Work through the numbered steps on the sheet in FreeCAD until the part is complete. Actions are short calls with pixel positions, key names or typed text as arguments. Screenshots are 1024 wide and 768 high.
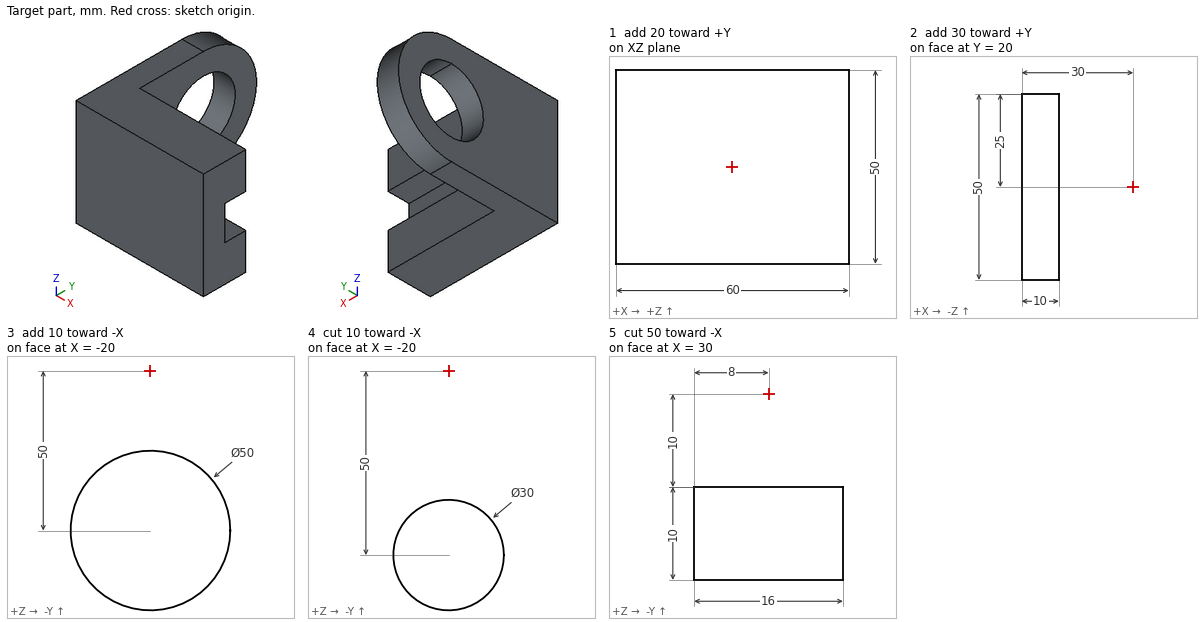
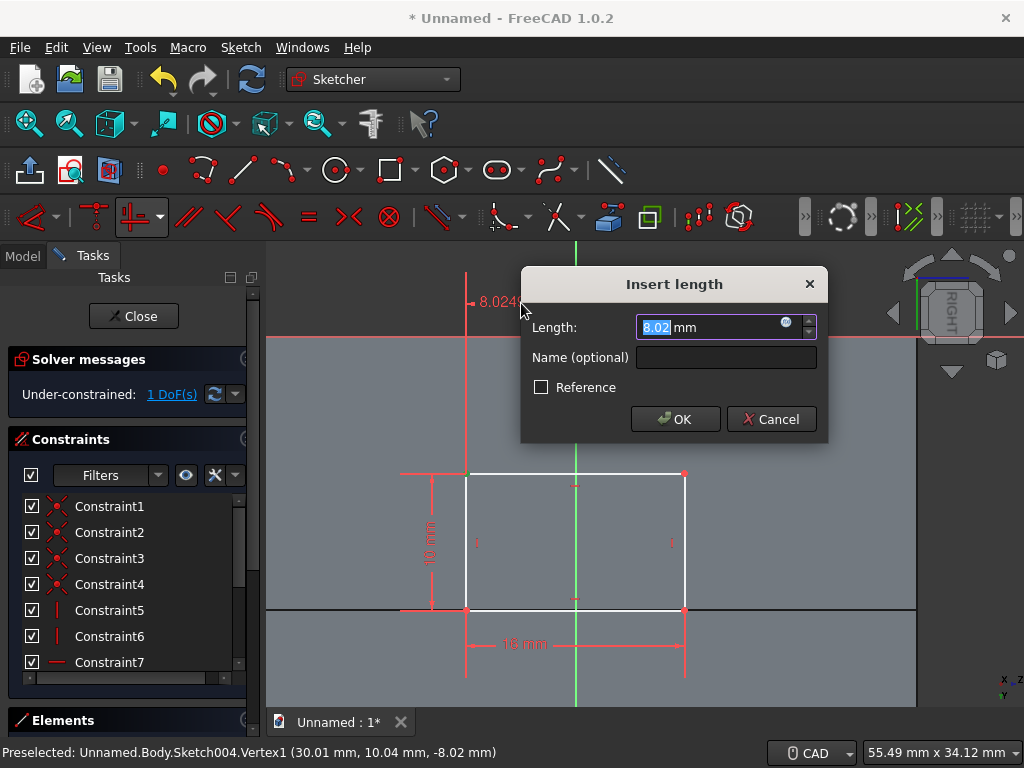
text(8)
key(Return)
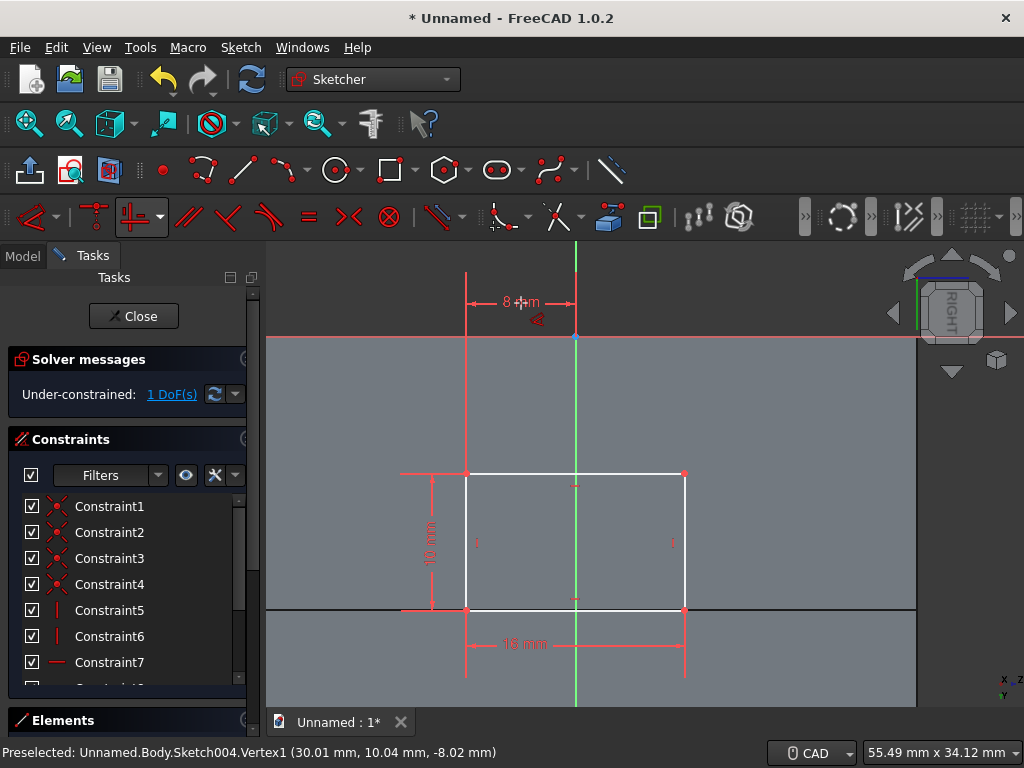
click(466, 474)
click(432, 405)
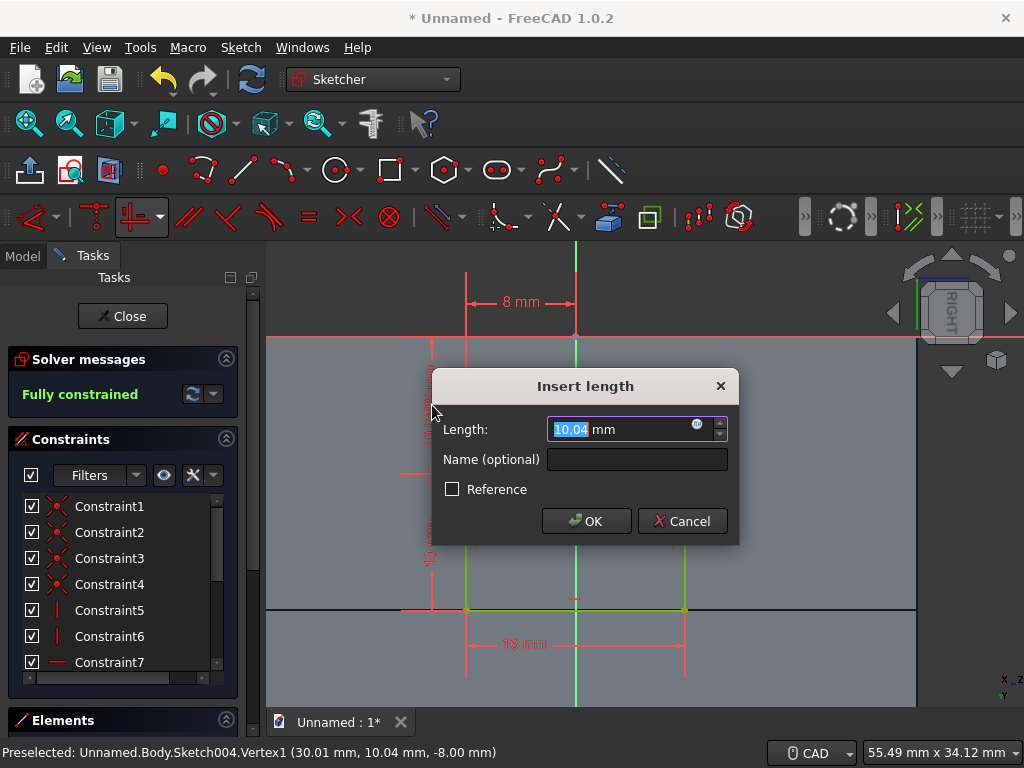
text(10)
key(Return)
key(Escape)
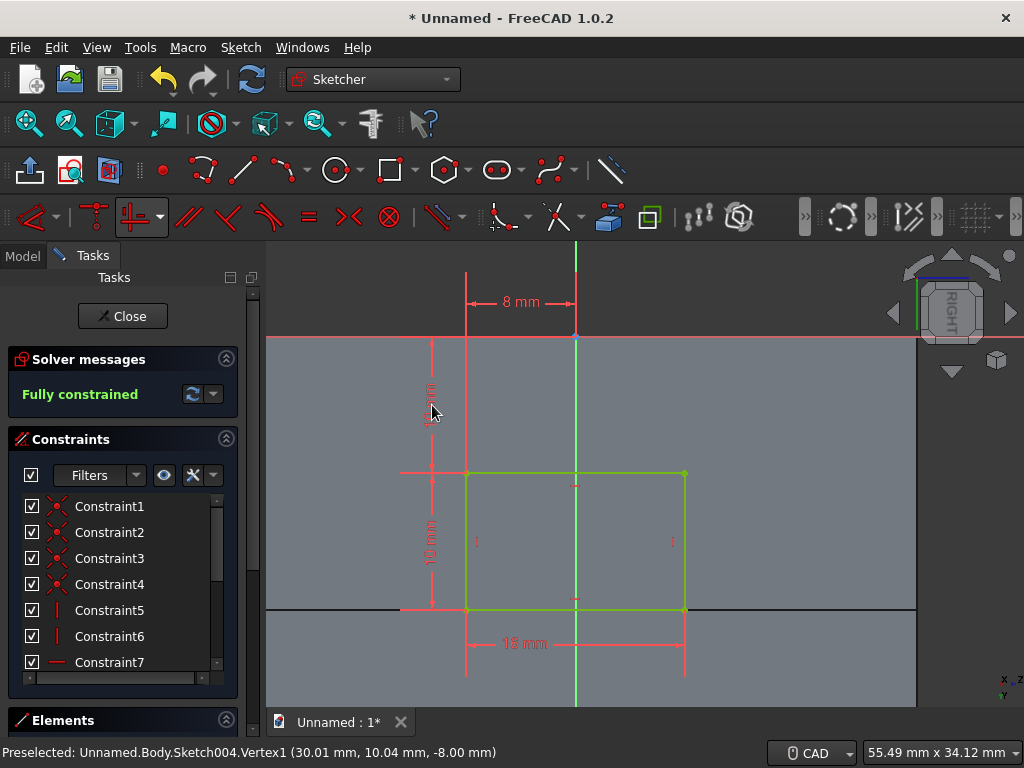
click(123, 316)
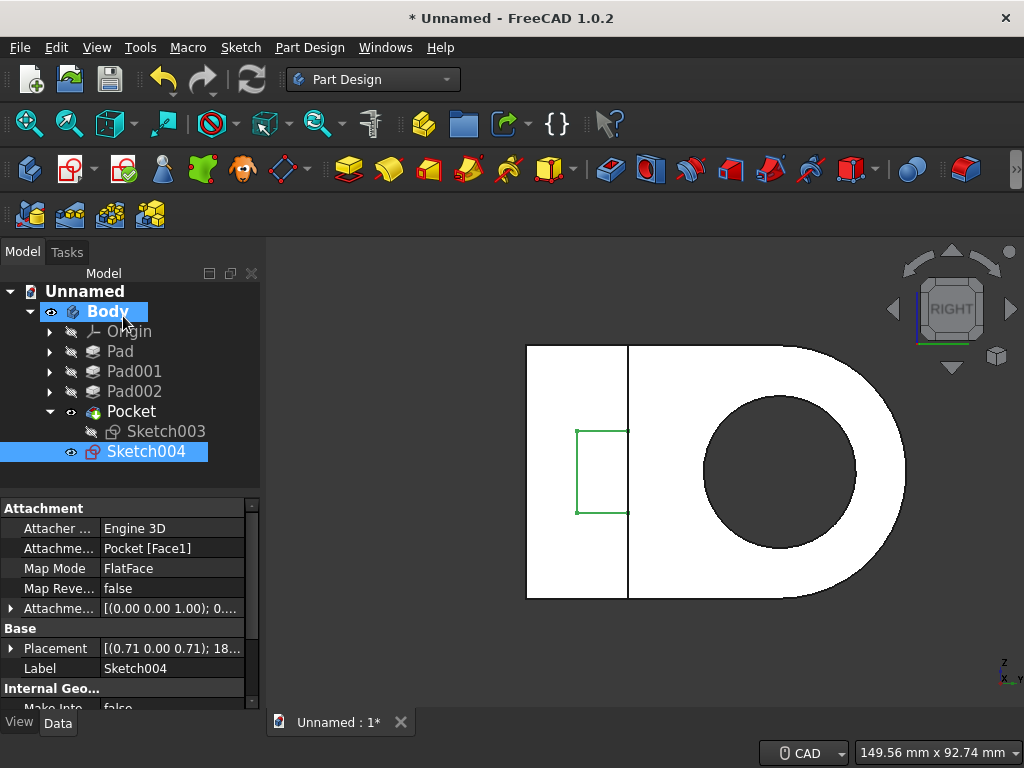
click(612, 170)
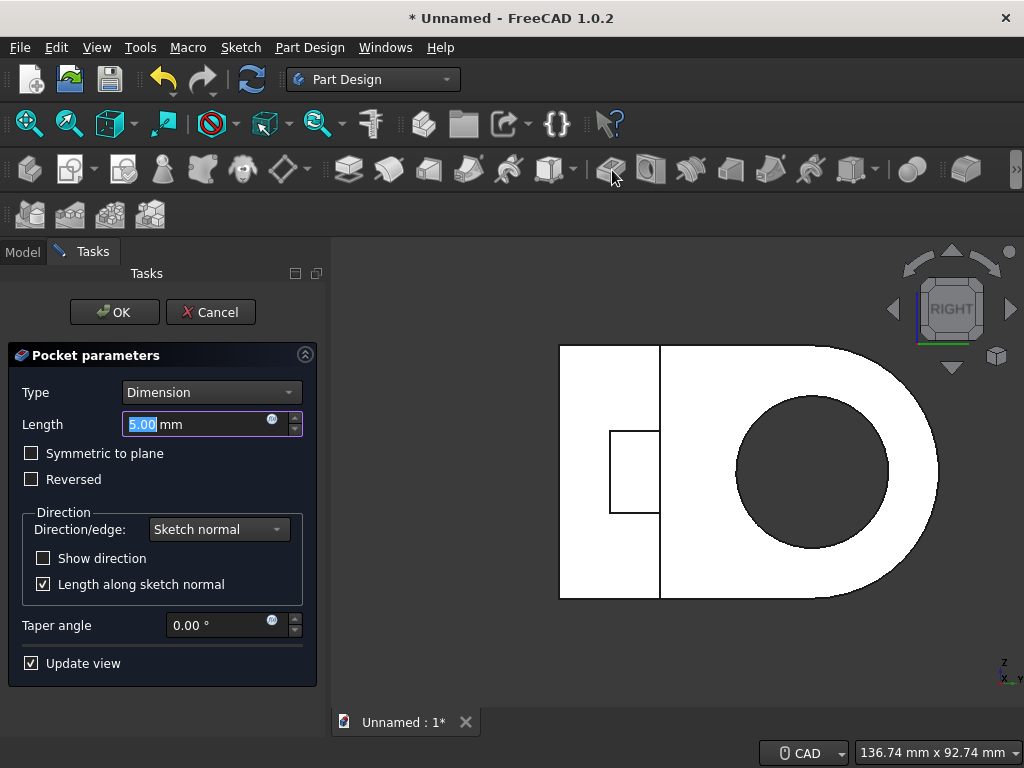
text(50)
key(Tab)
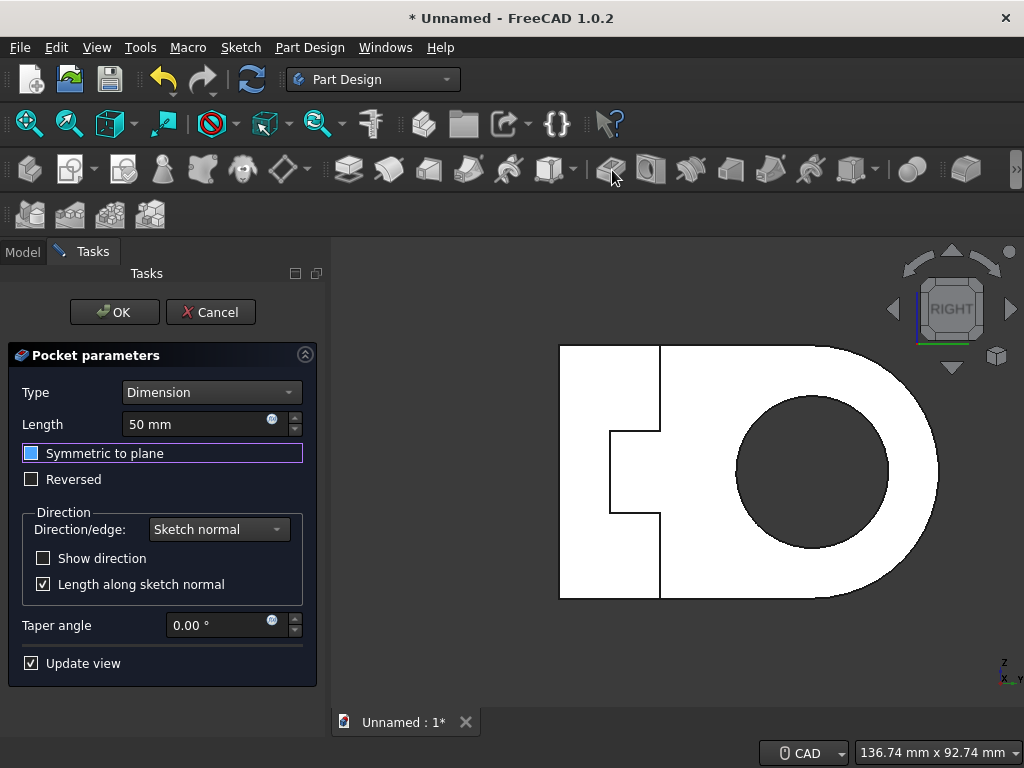
click(115, 312)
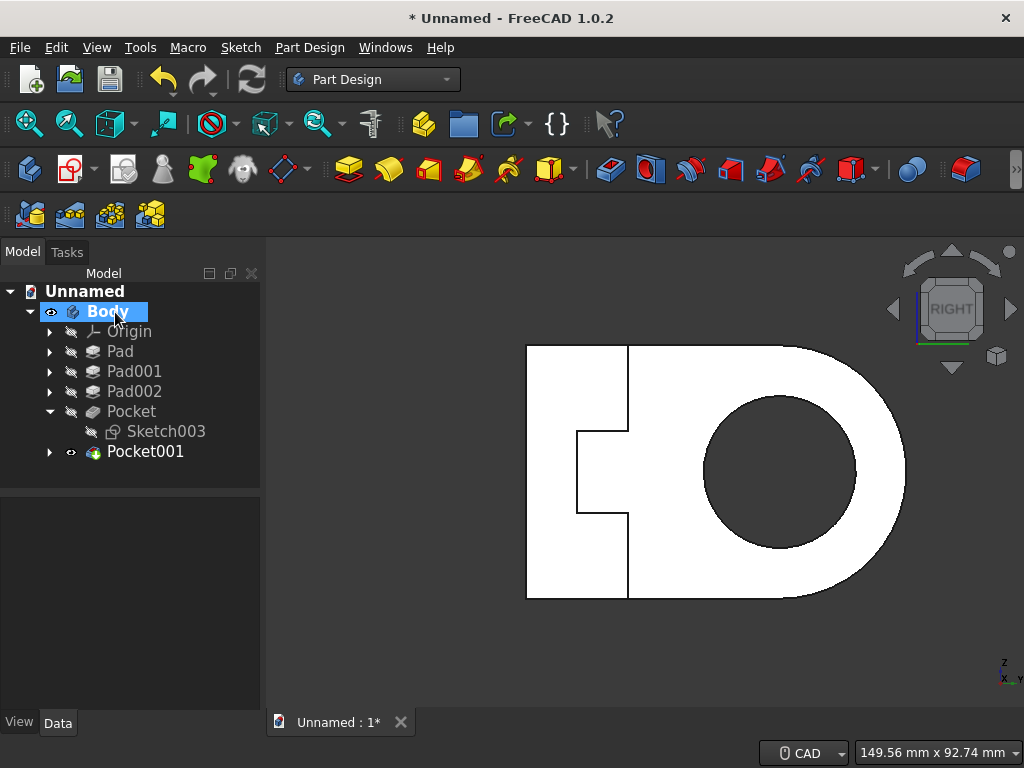
key(0)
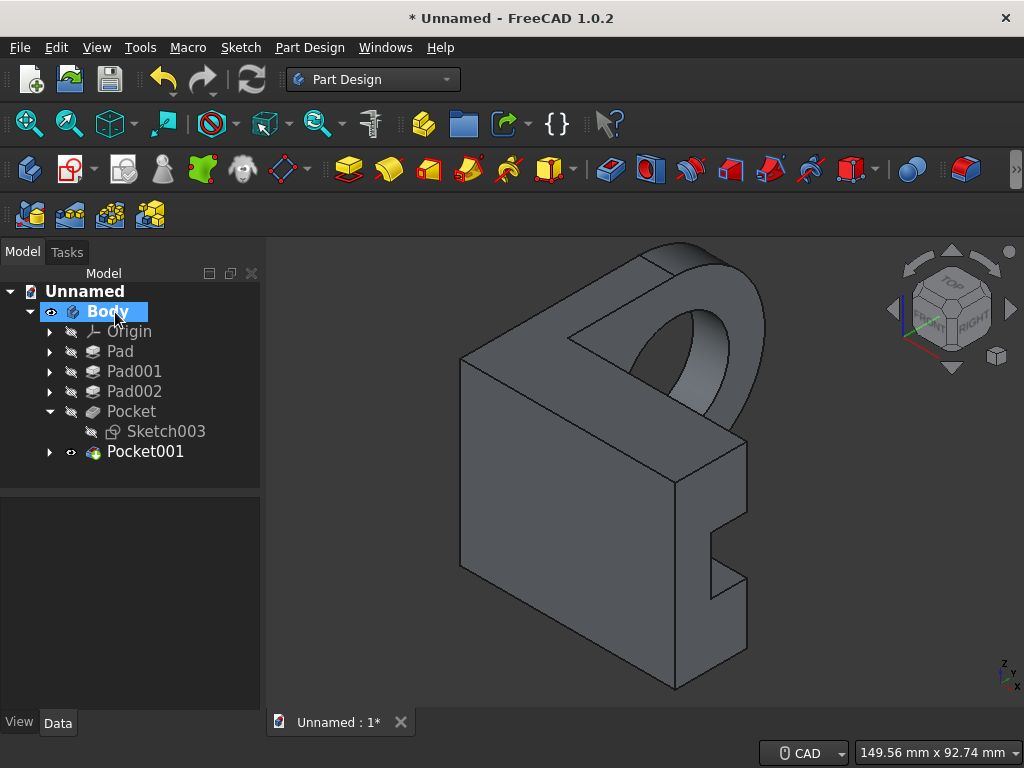
click(30, 124)